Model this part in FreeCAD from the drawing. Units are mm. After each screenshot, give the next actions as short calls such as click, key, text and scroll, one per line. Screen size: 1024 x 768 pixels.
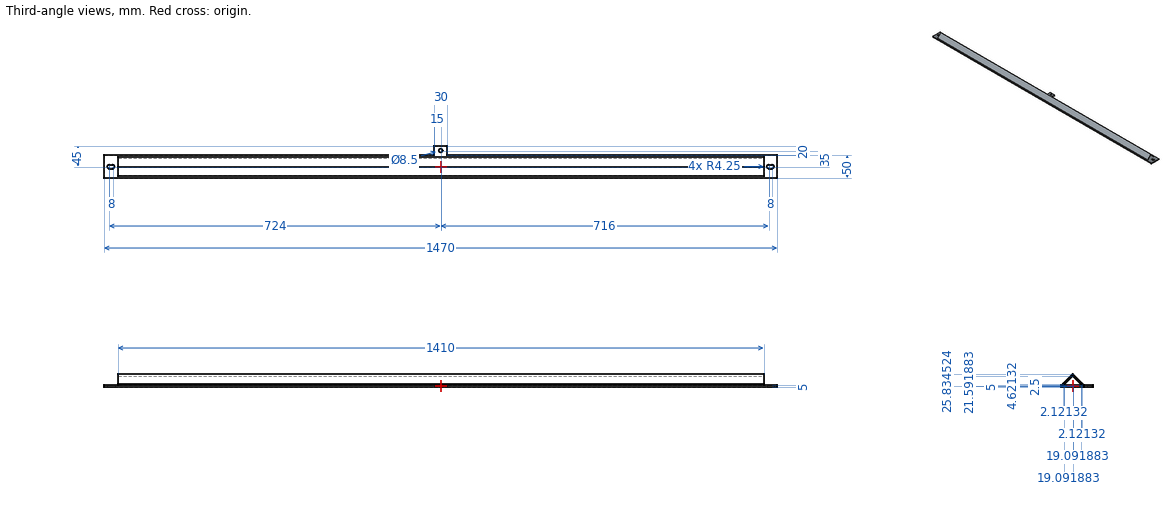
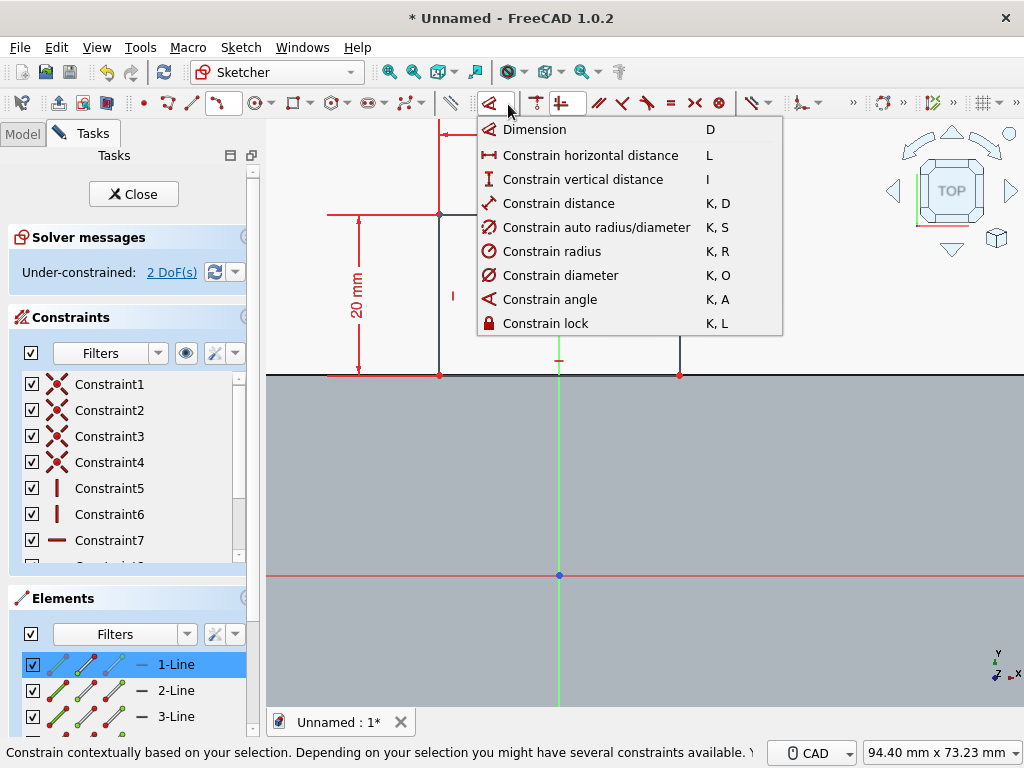
click(630, 155)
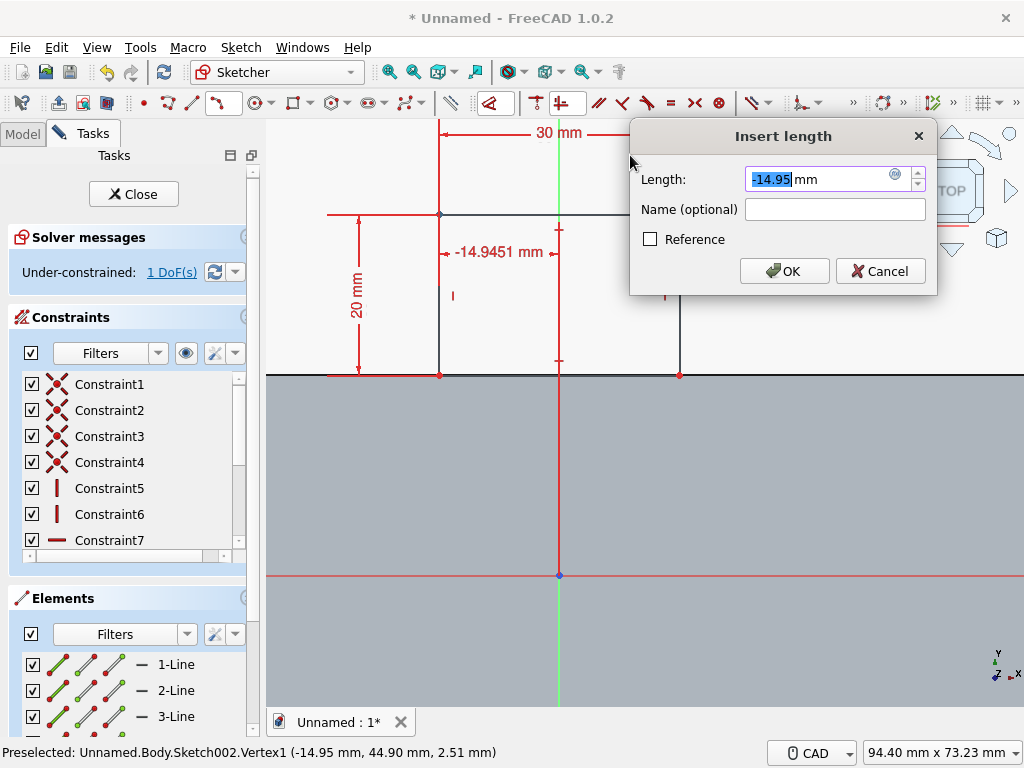
text(-15)
key(Return)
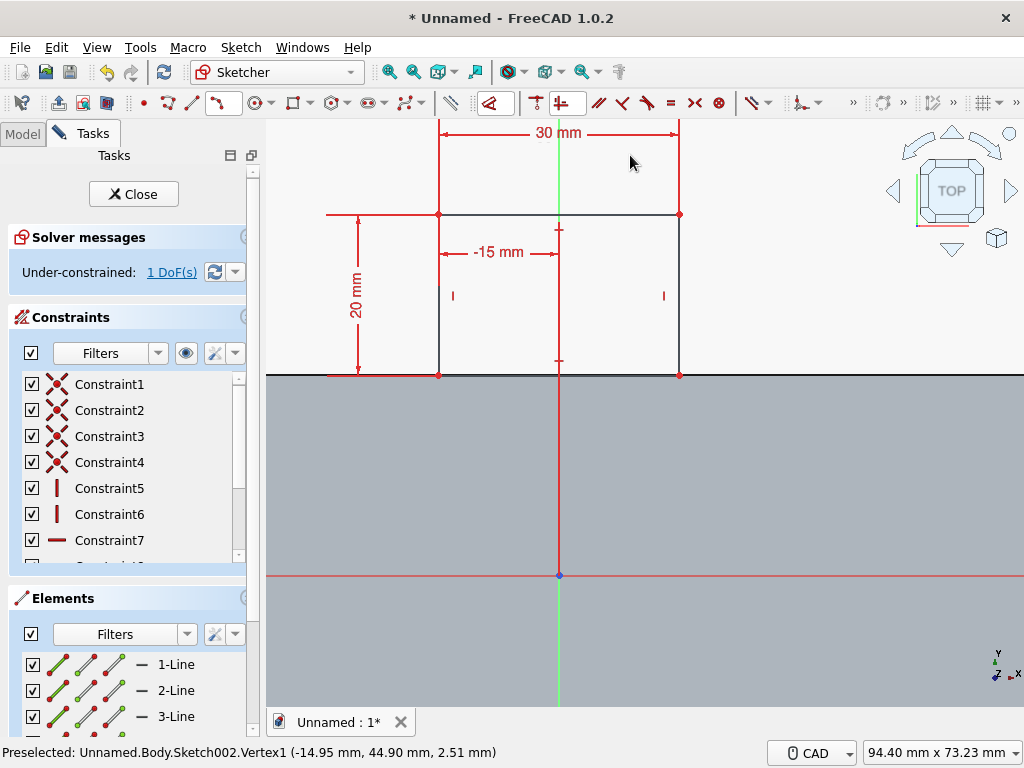
click(439, 215)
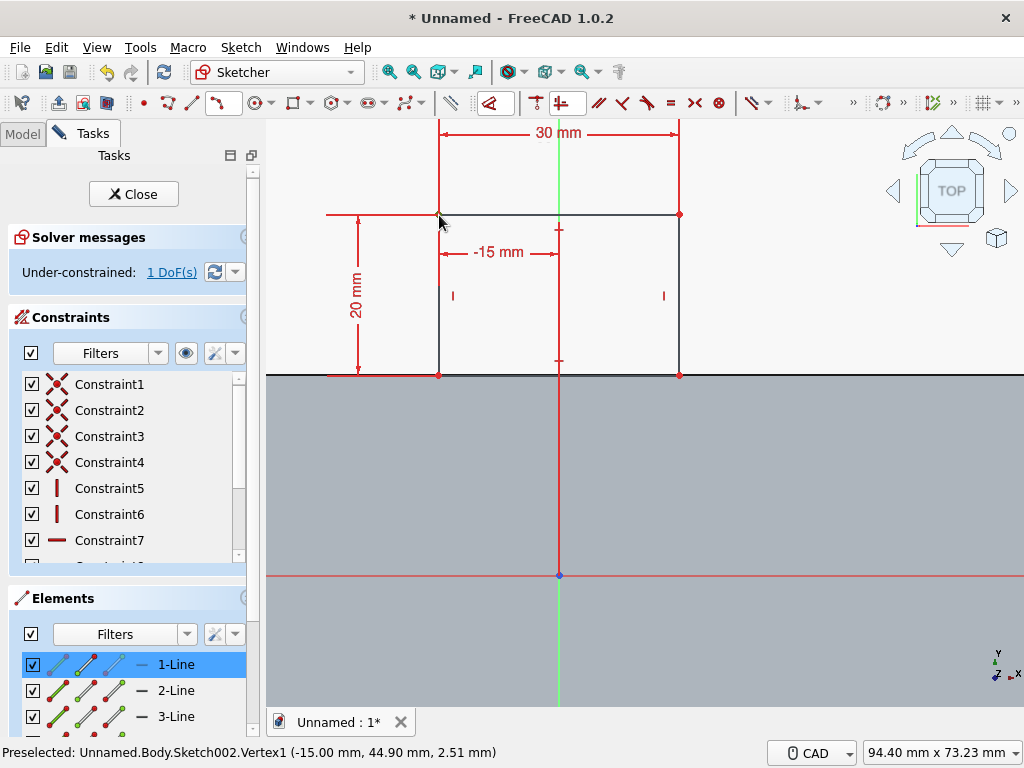
click(508, 104)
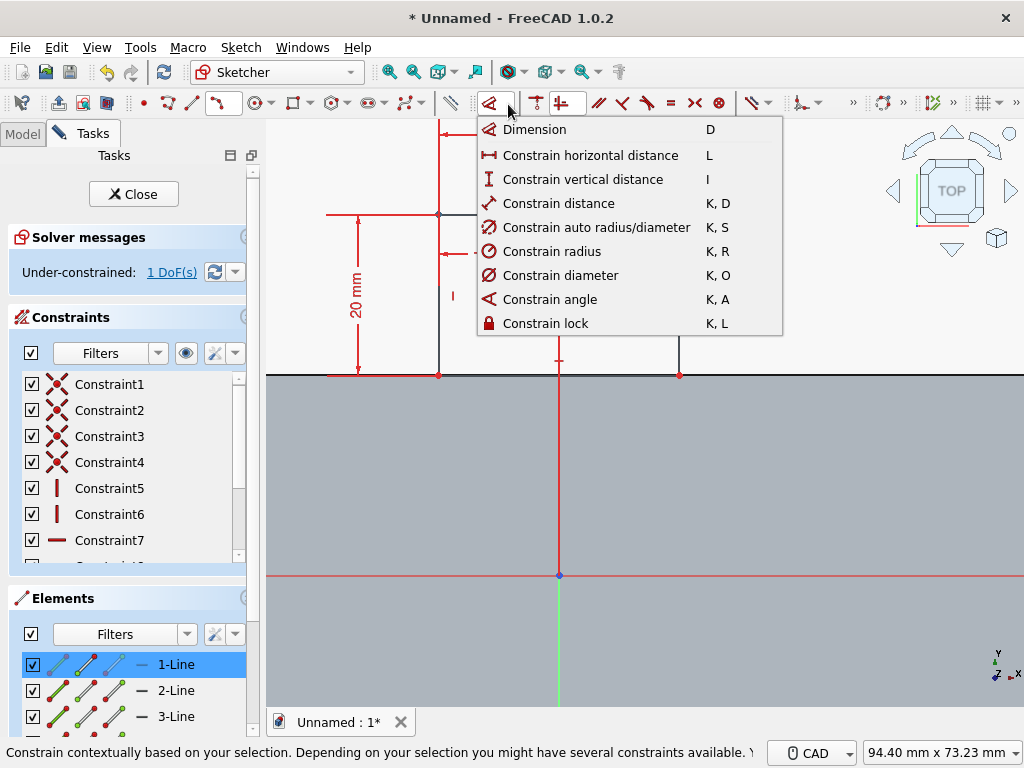
click(630, 179)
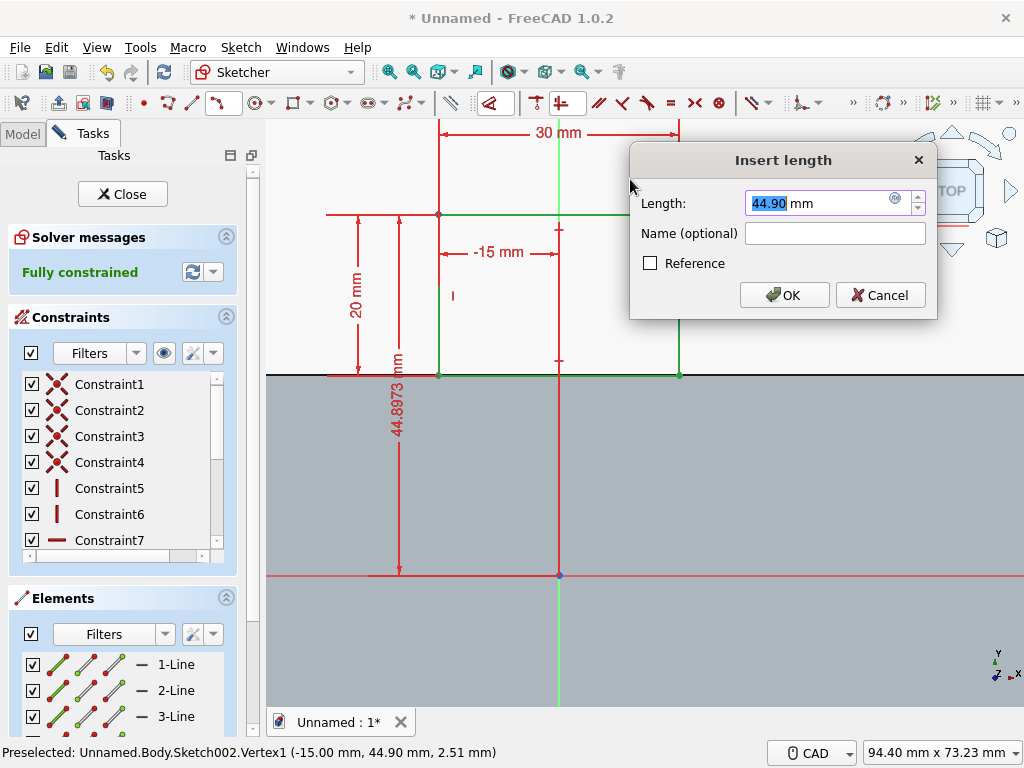
text(45)
key(Return)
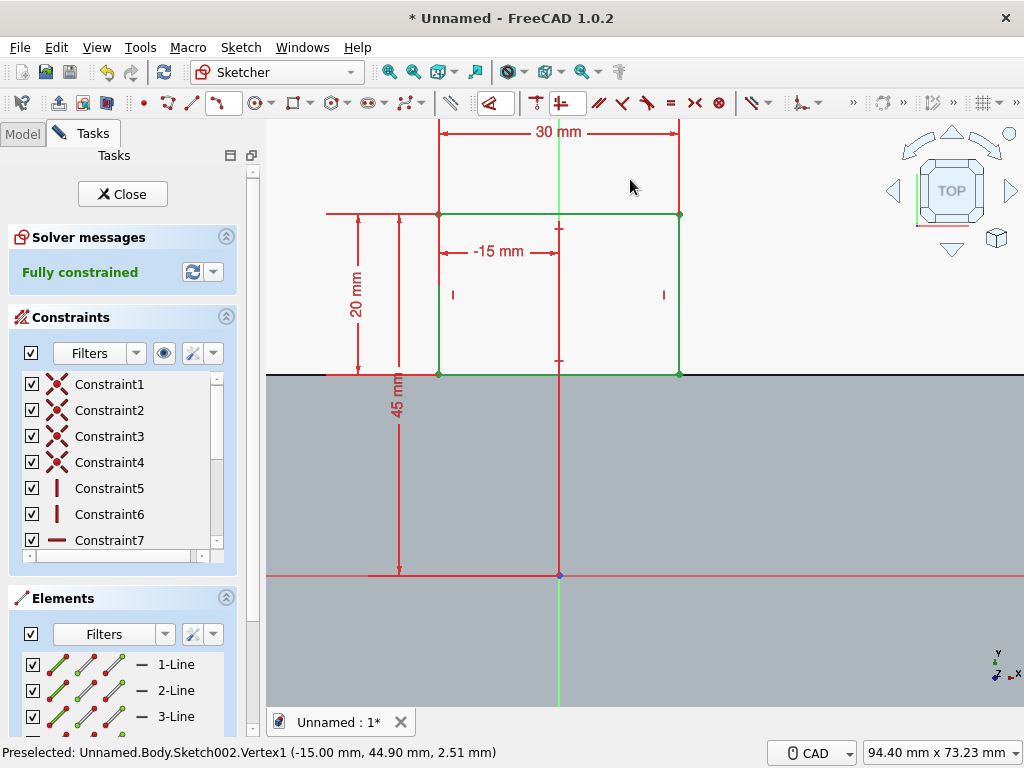
click(123, 194)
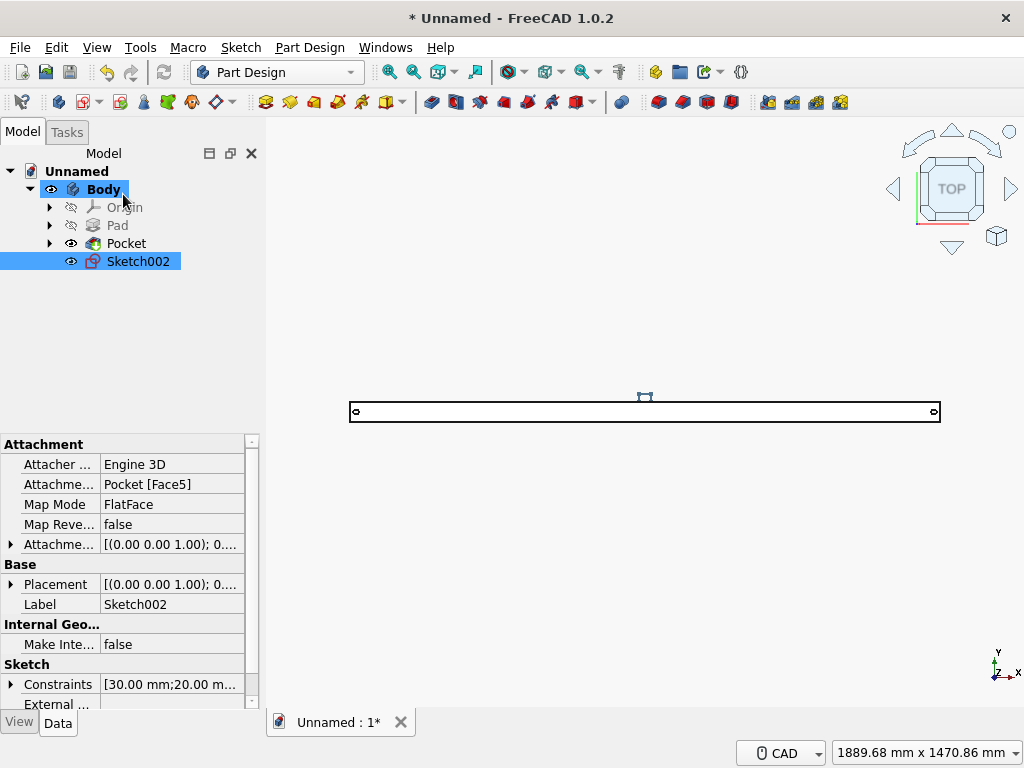
click(266, 102)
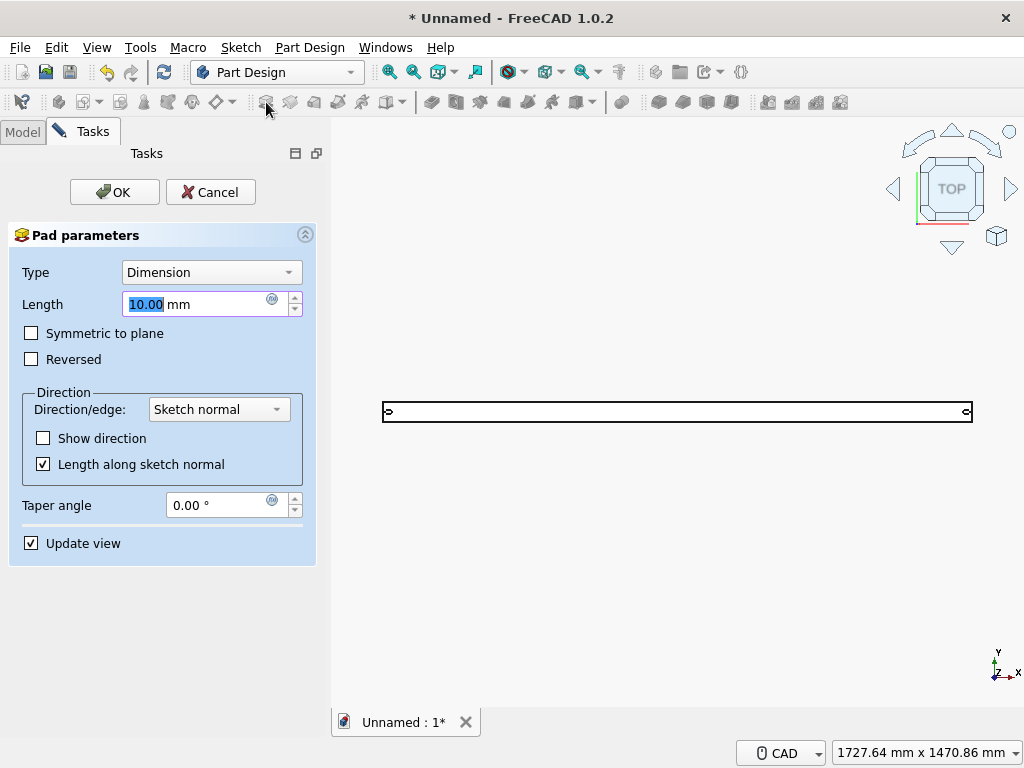
text(5)
key(Tab)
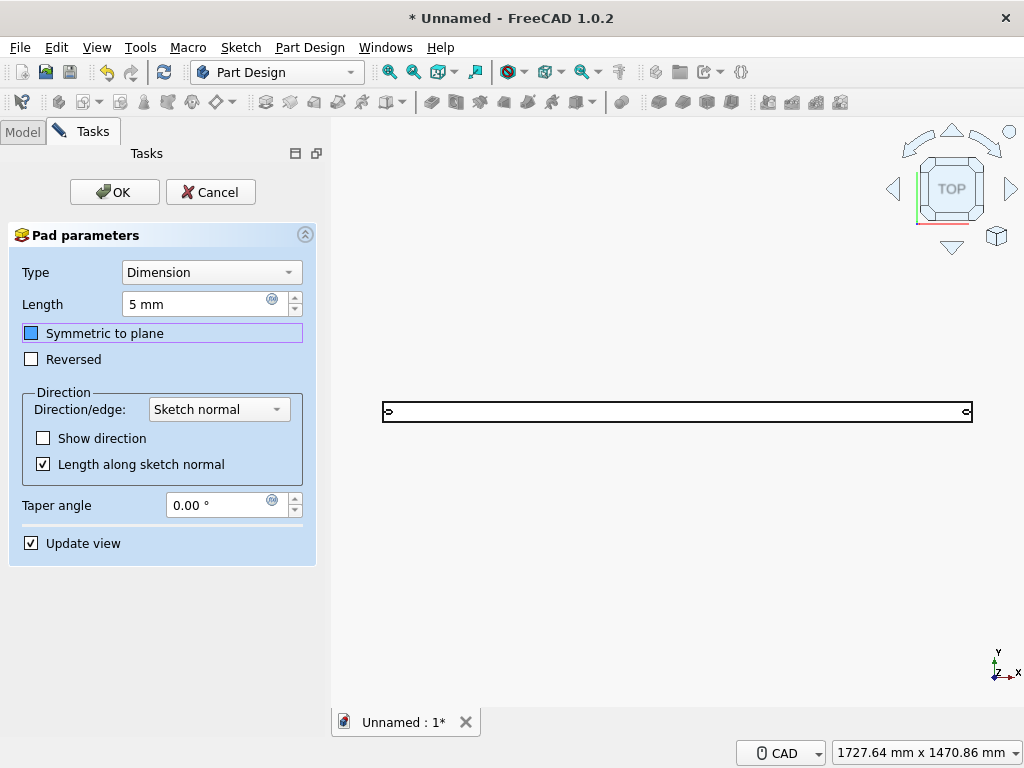
click(30, 359)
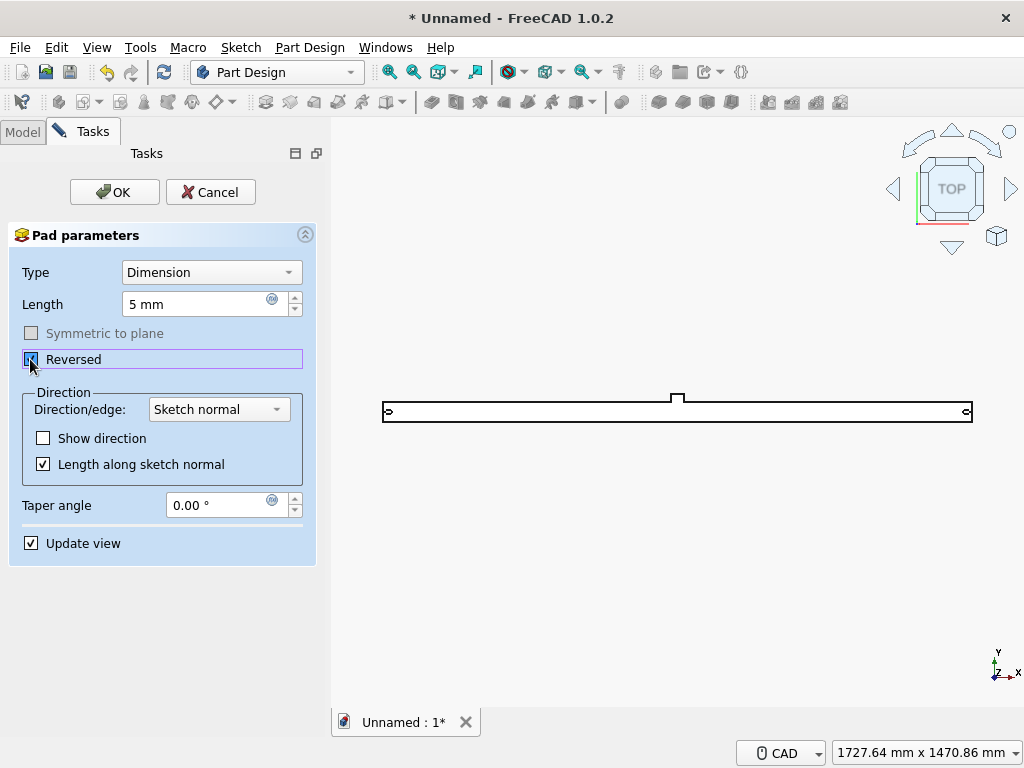
click(115, 192)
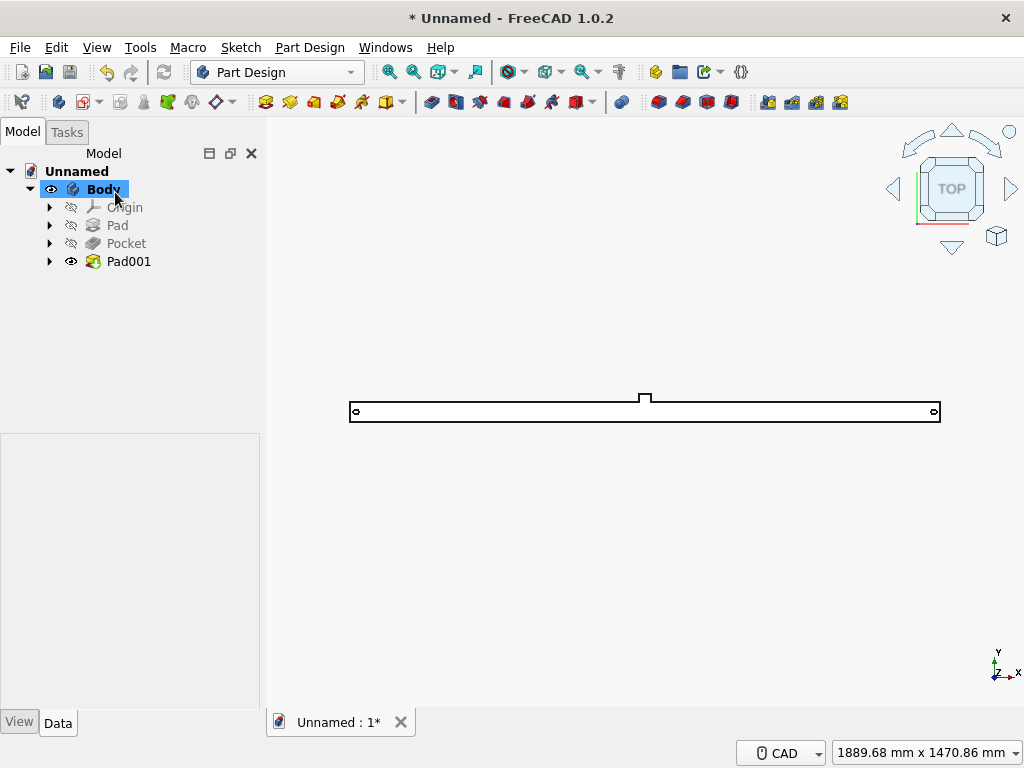
click(898, 411)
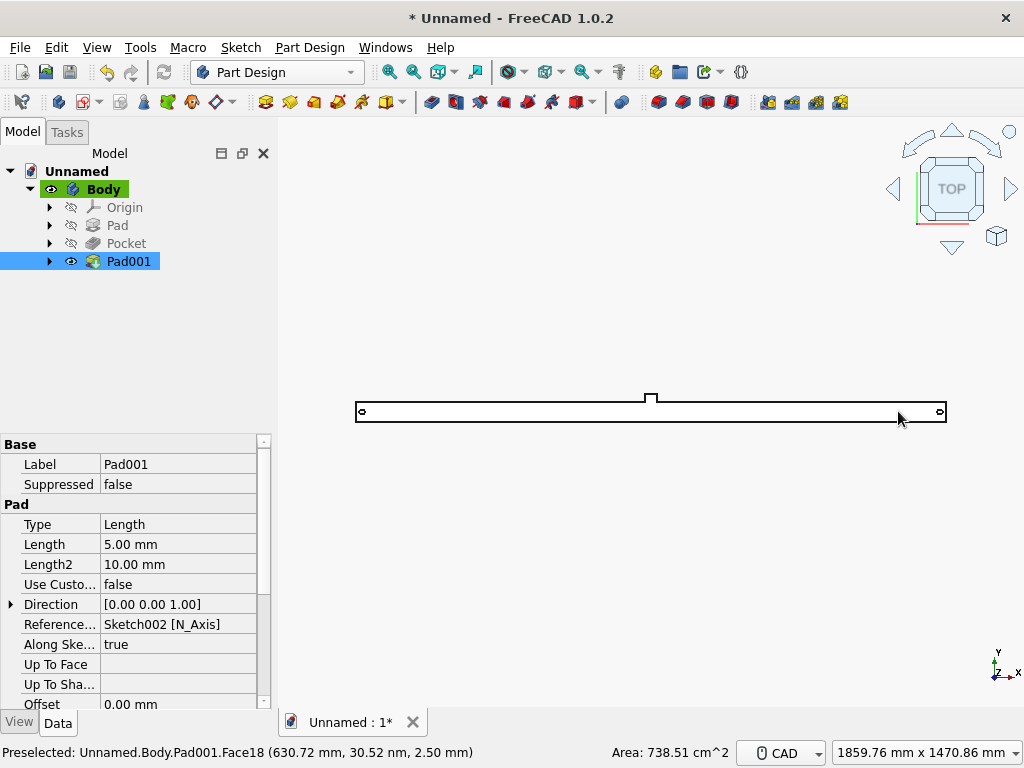
click(84, 102)